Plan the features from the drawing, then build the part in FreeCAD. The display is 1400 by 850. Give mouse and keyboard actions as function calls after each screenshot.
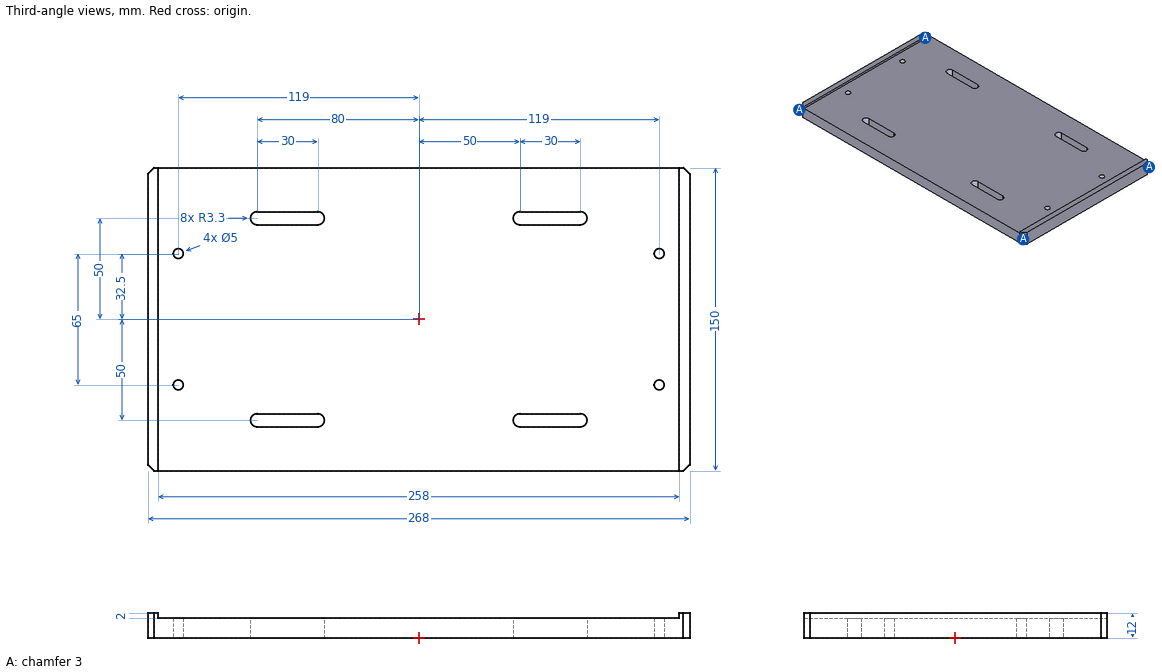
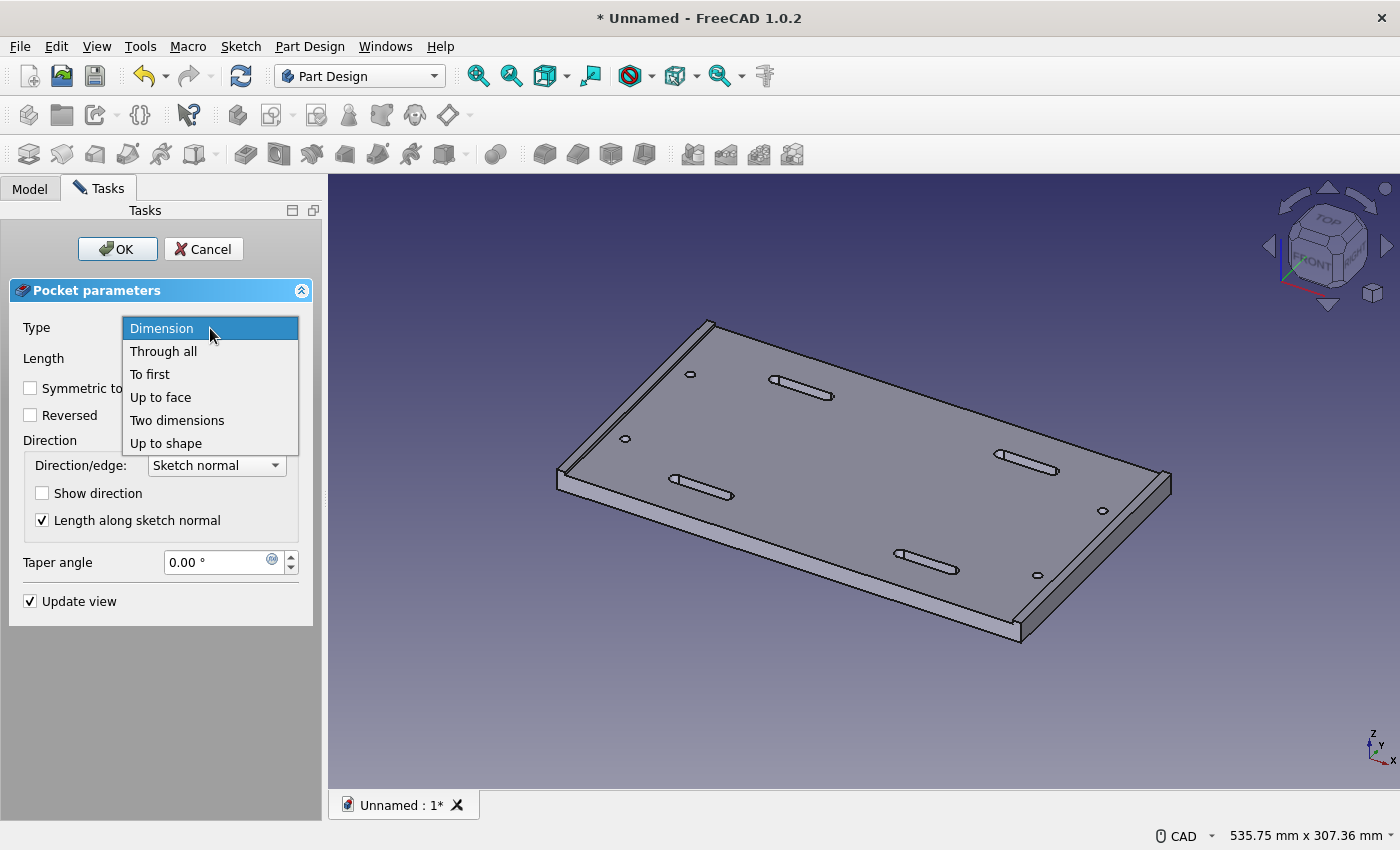
click(208, 352)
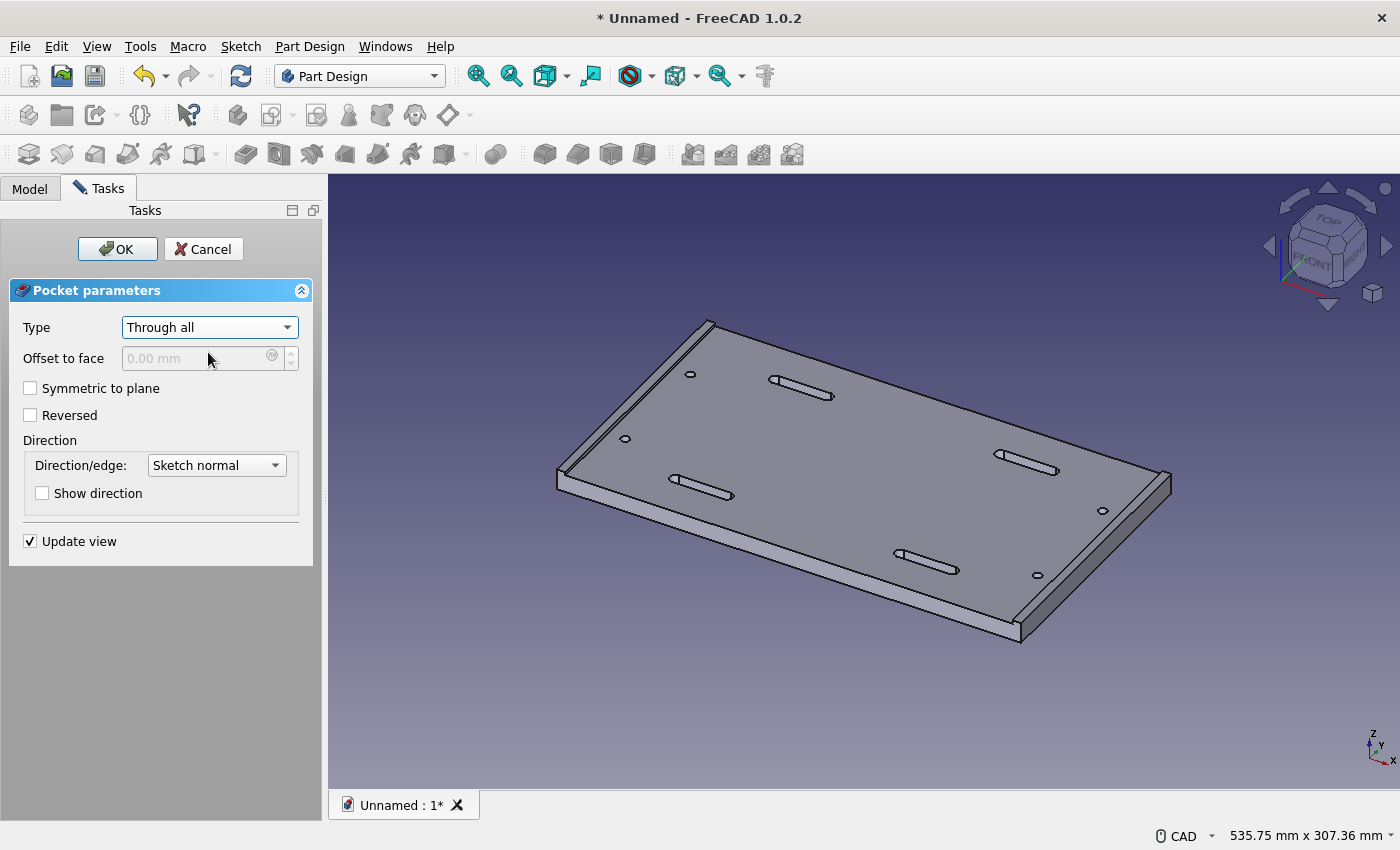
click(118, 249)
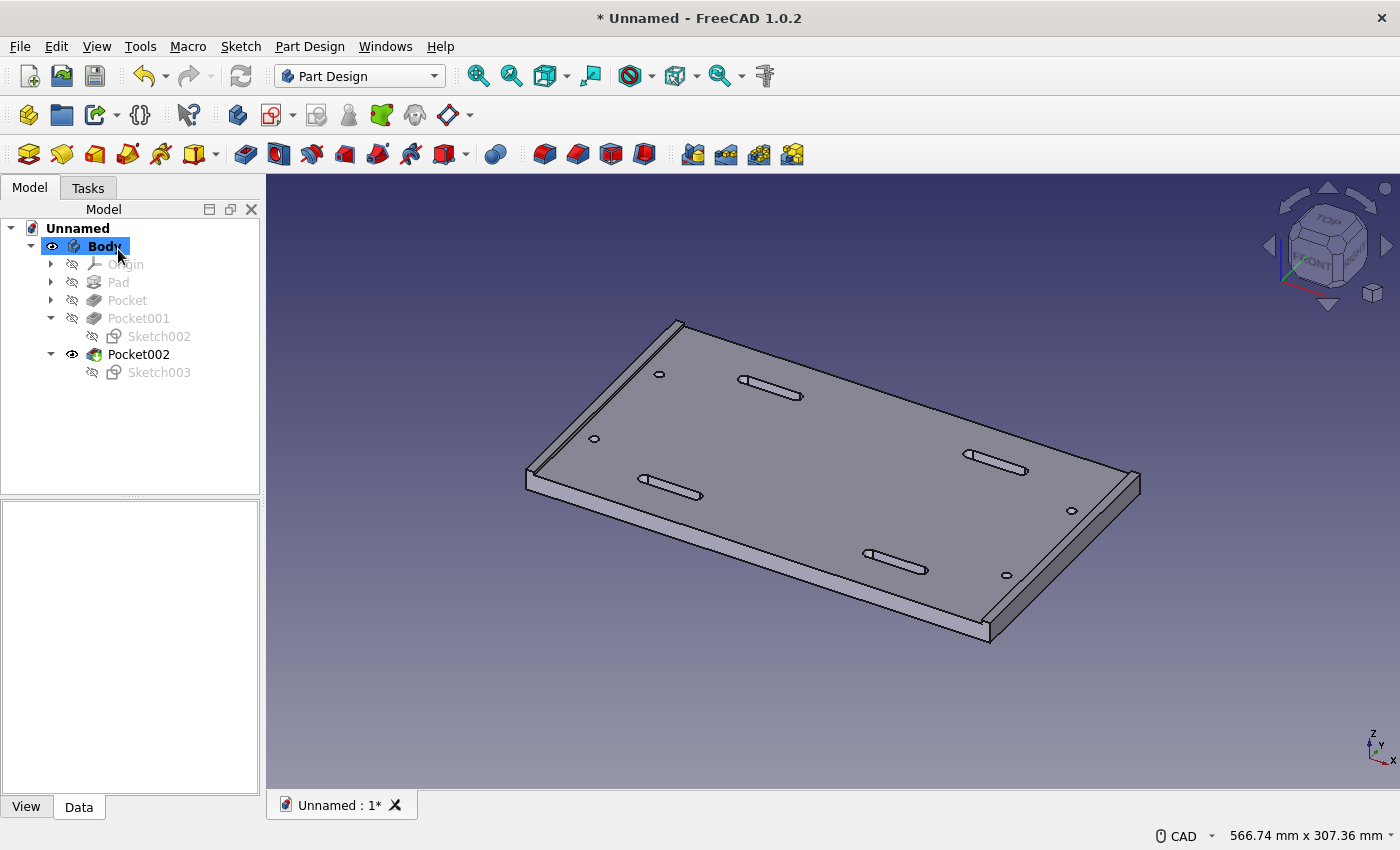
click(990, 632)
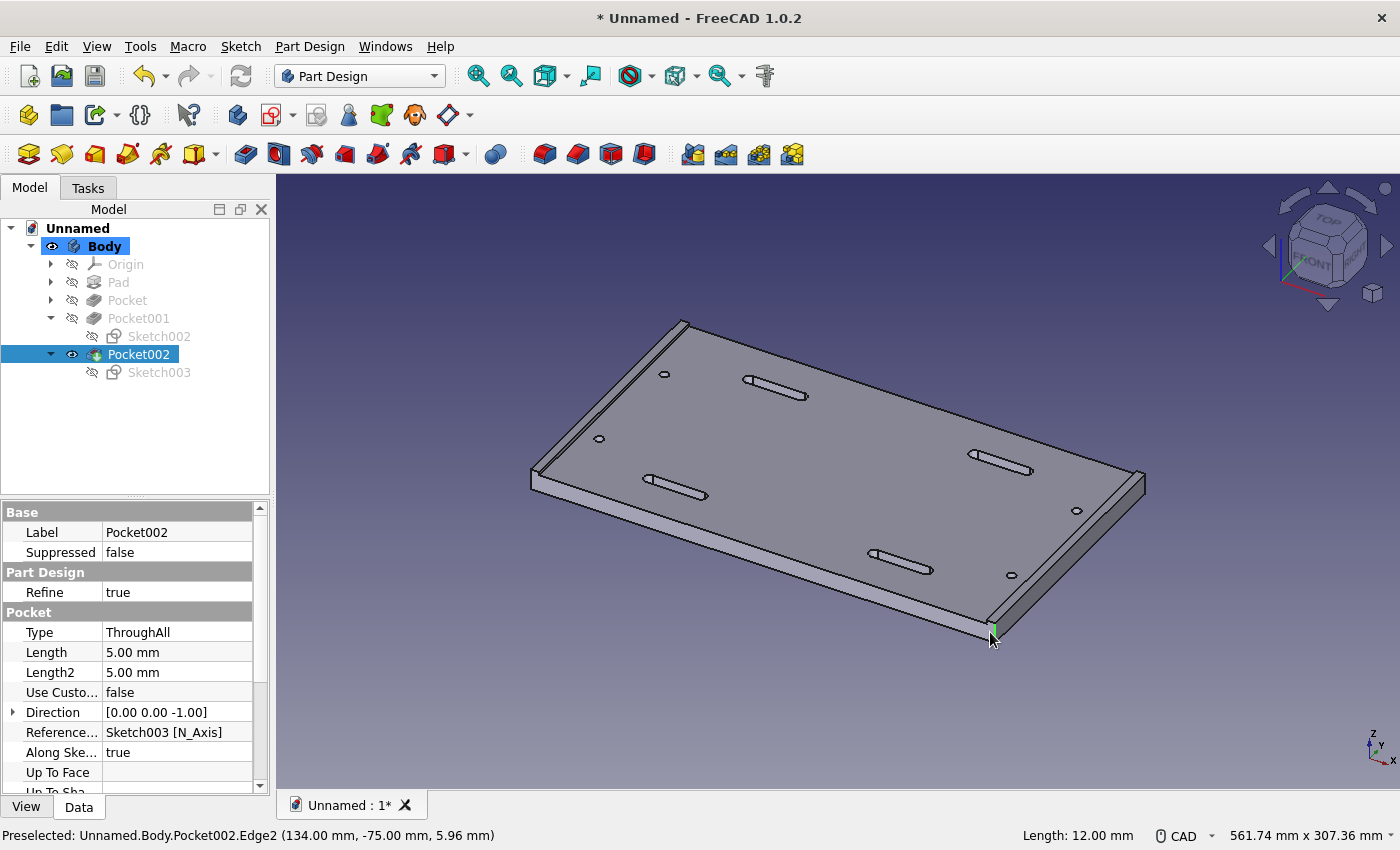
key(0)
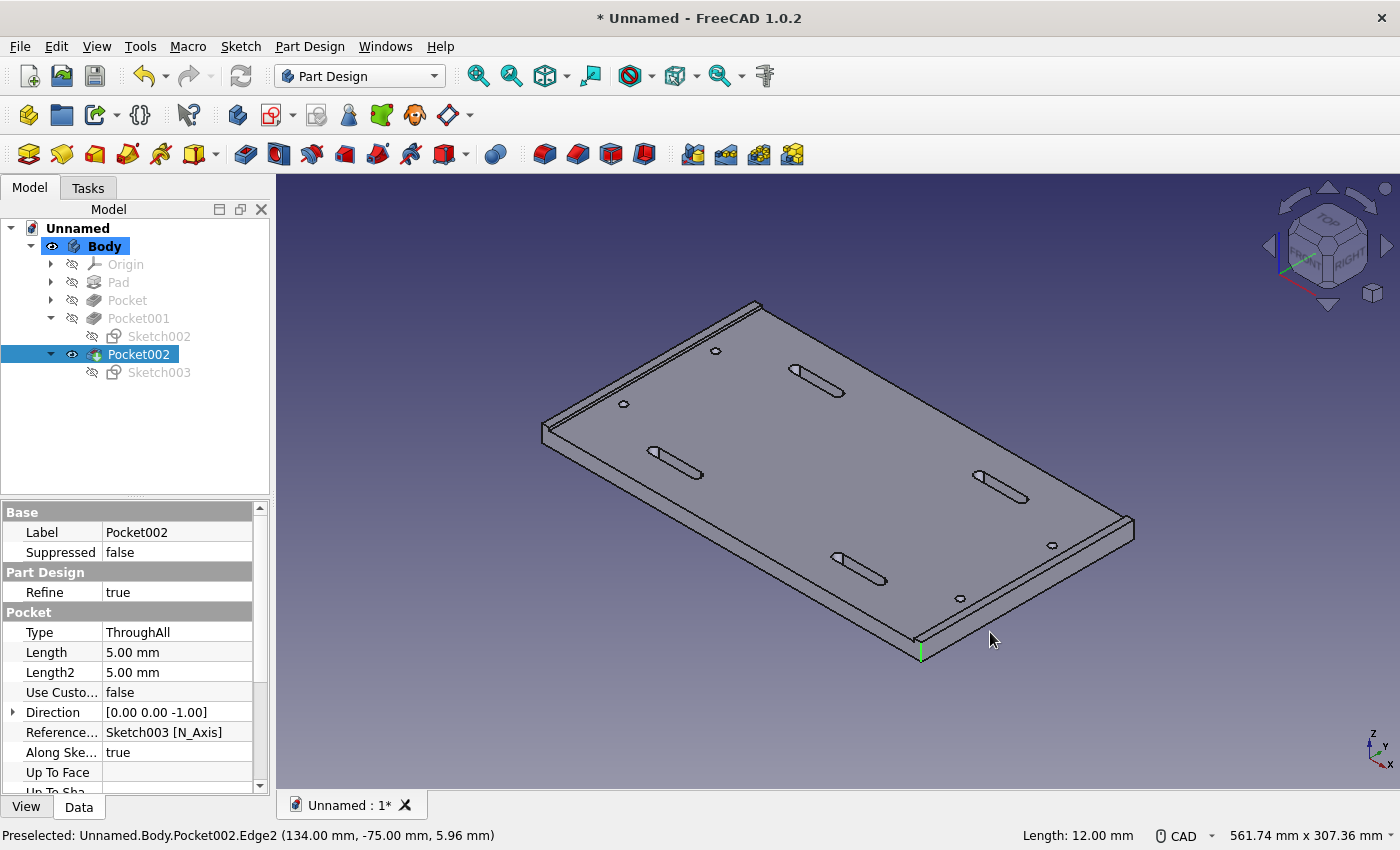
key(2)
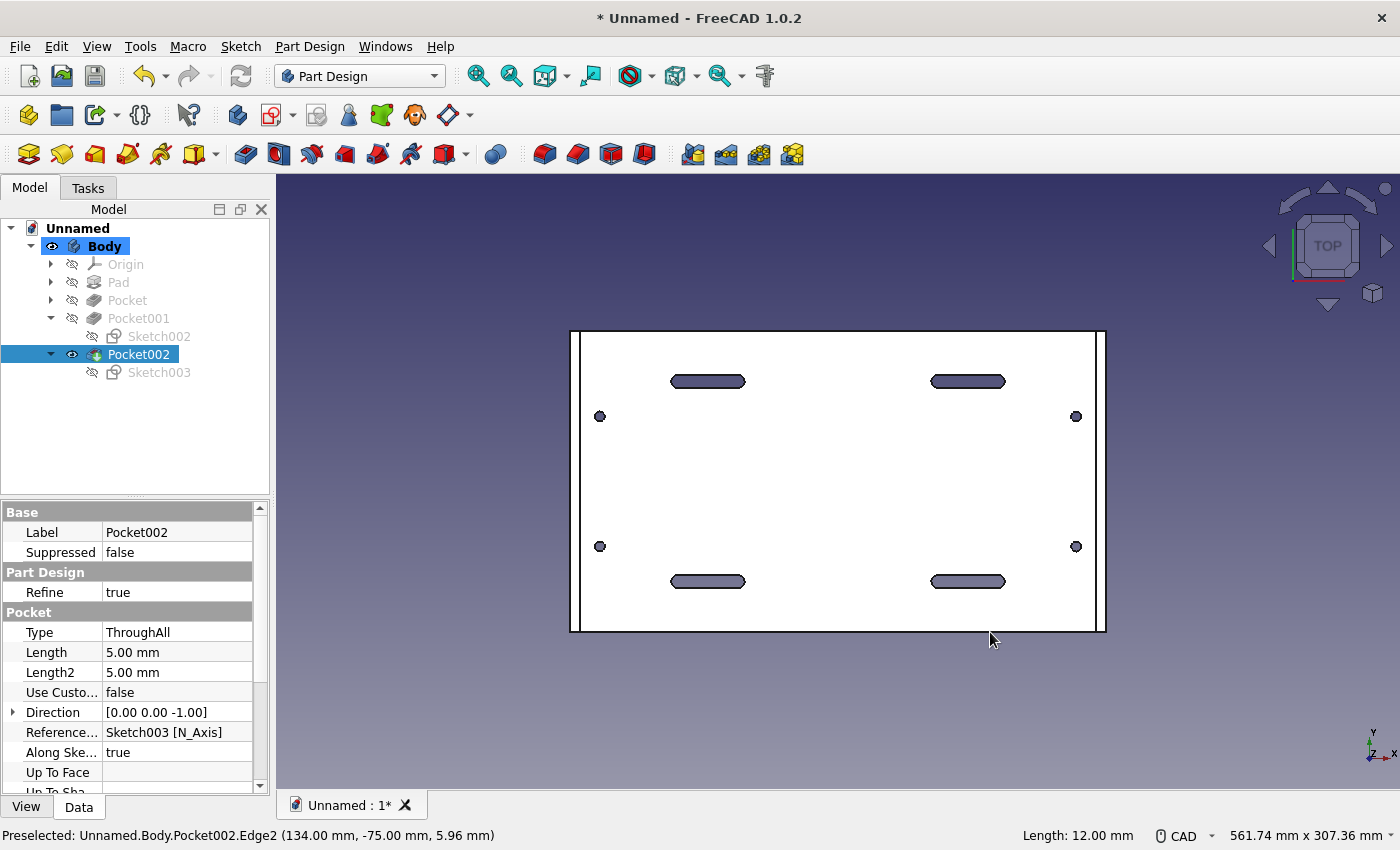
key(1)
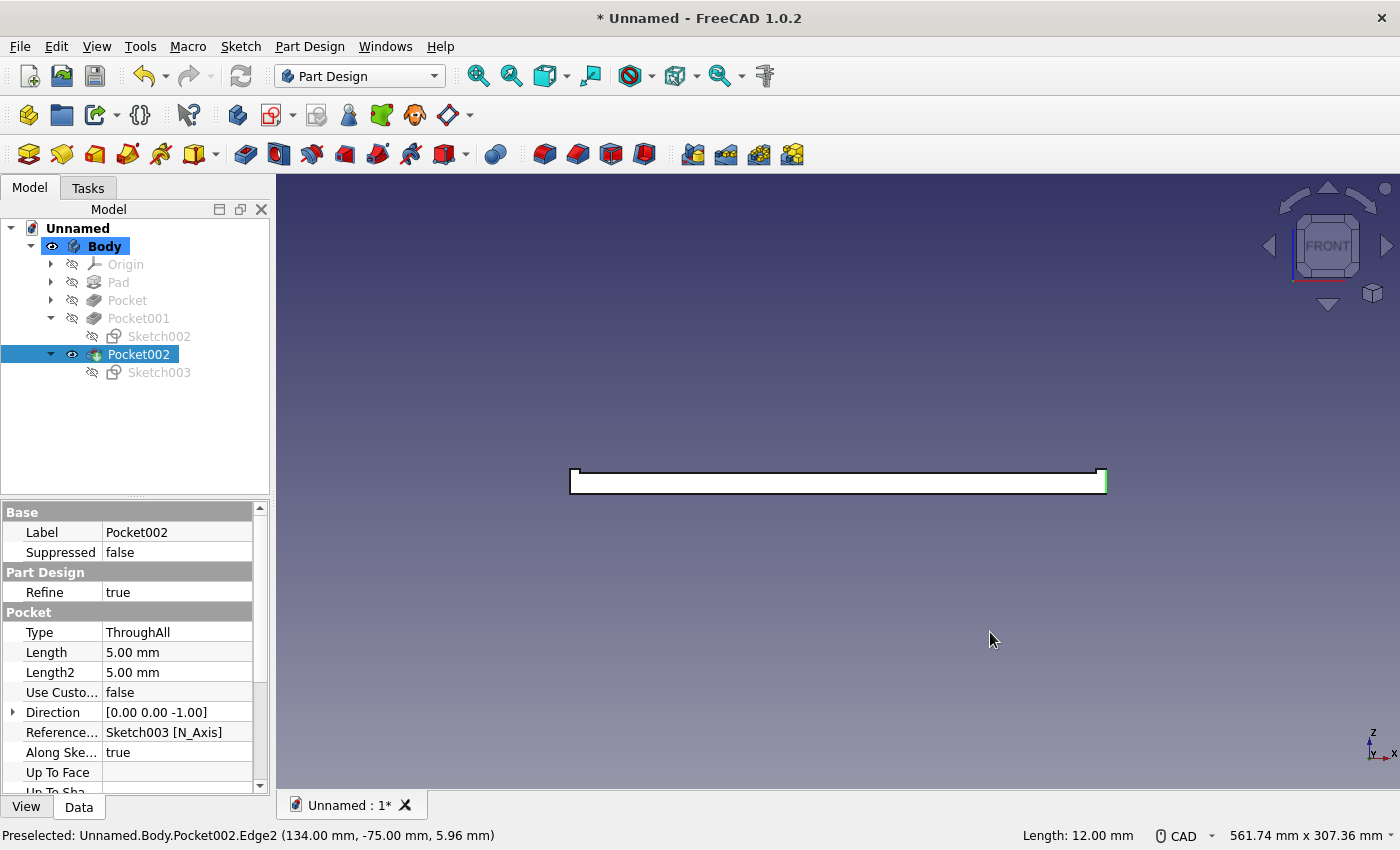
click(570, 480, ctrl)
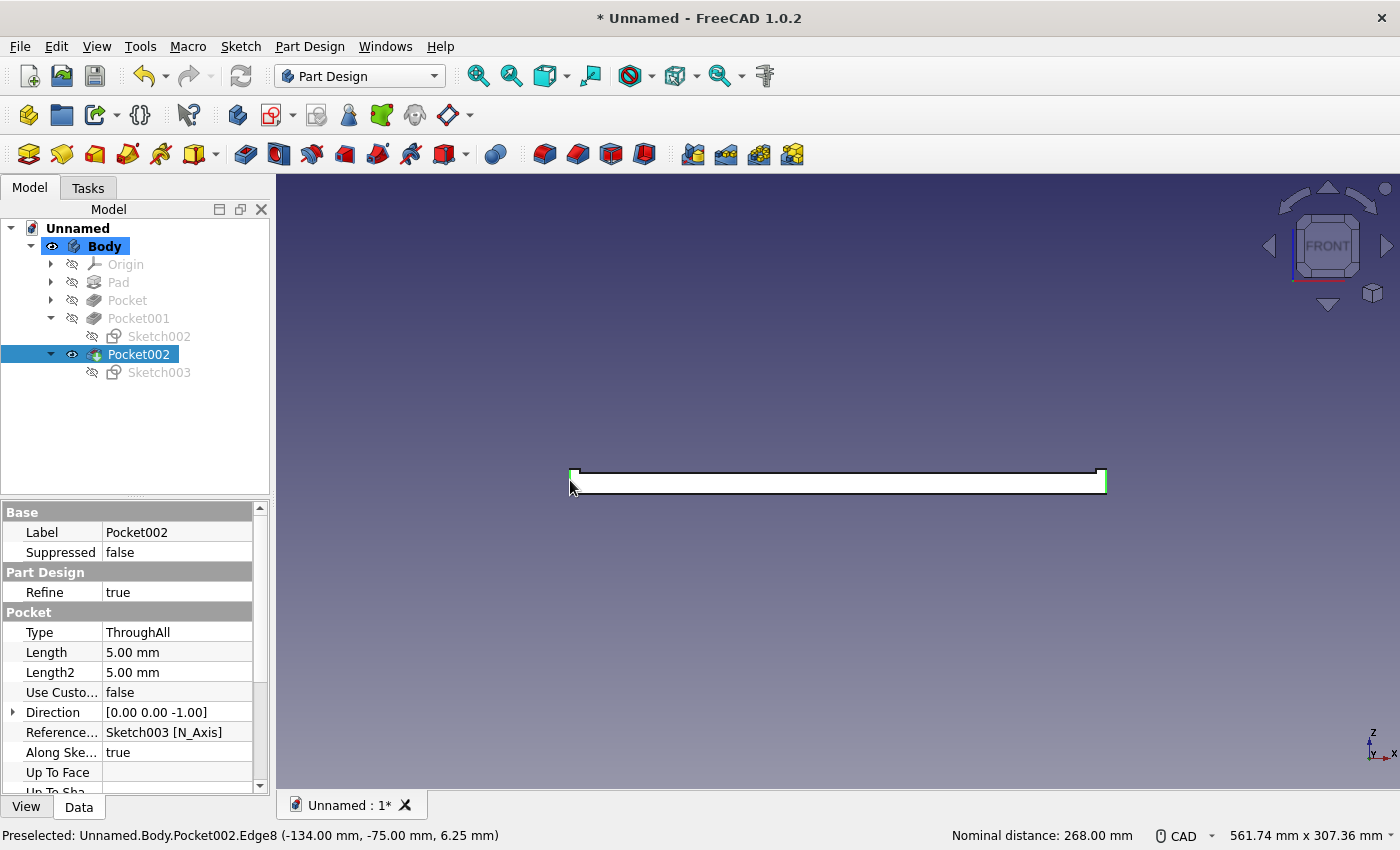
key(3)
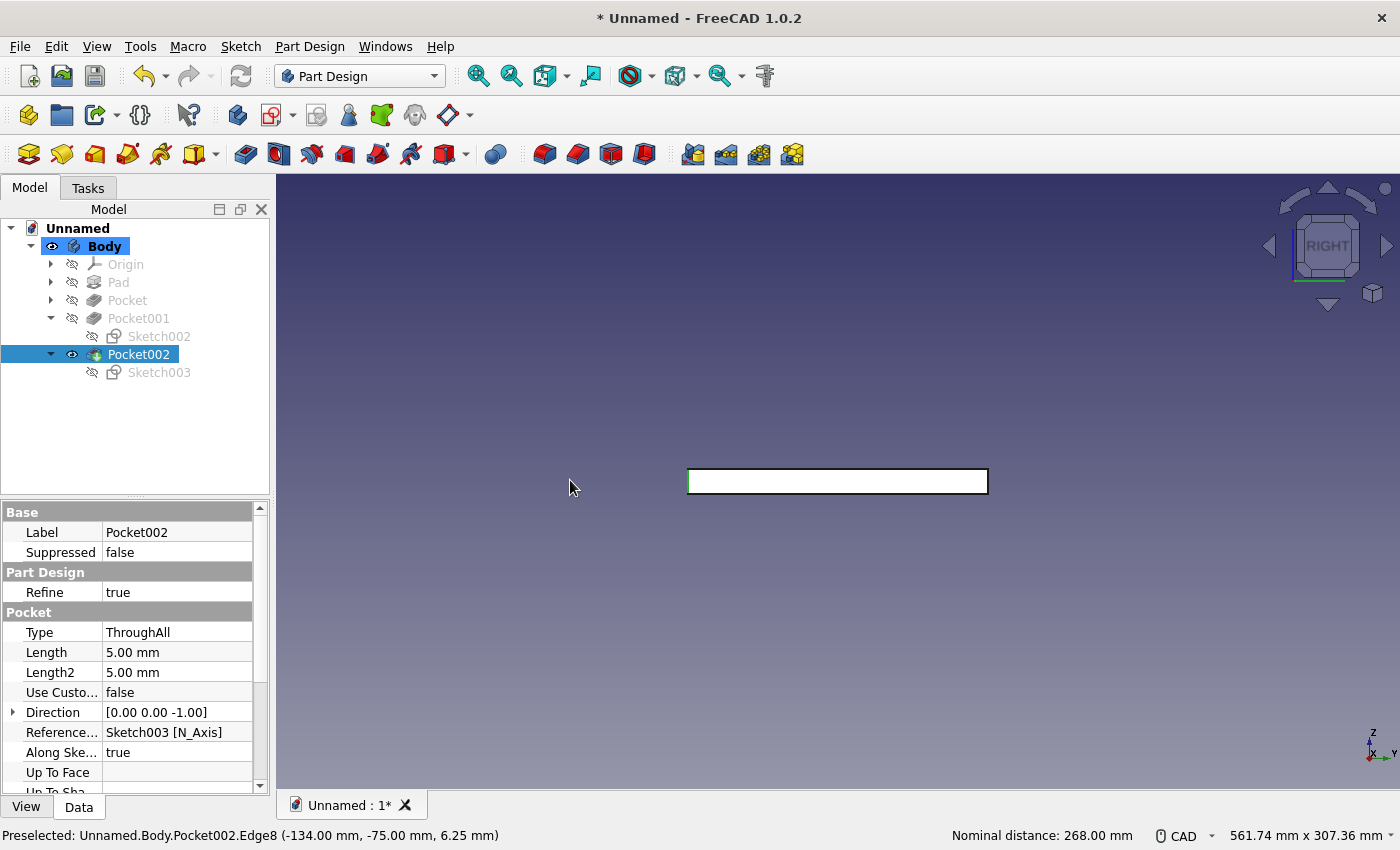
click(479, 76)